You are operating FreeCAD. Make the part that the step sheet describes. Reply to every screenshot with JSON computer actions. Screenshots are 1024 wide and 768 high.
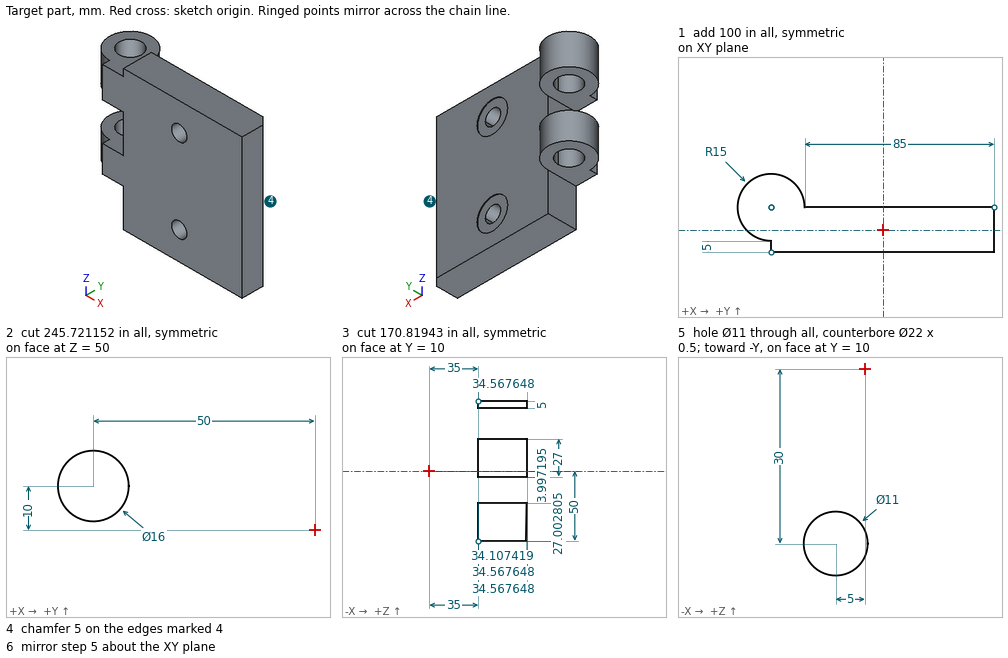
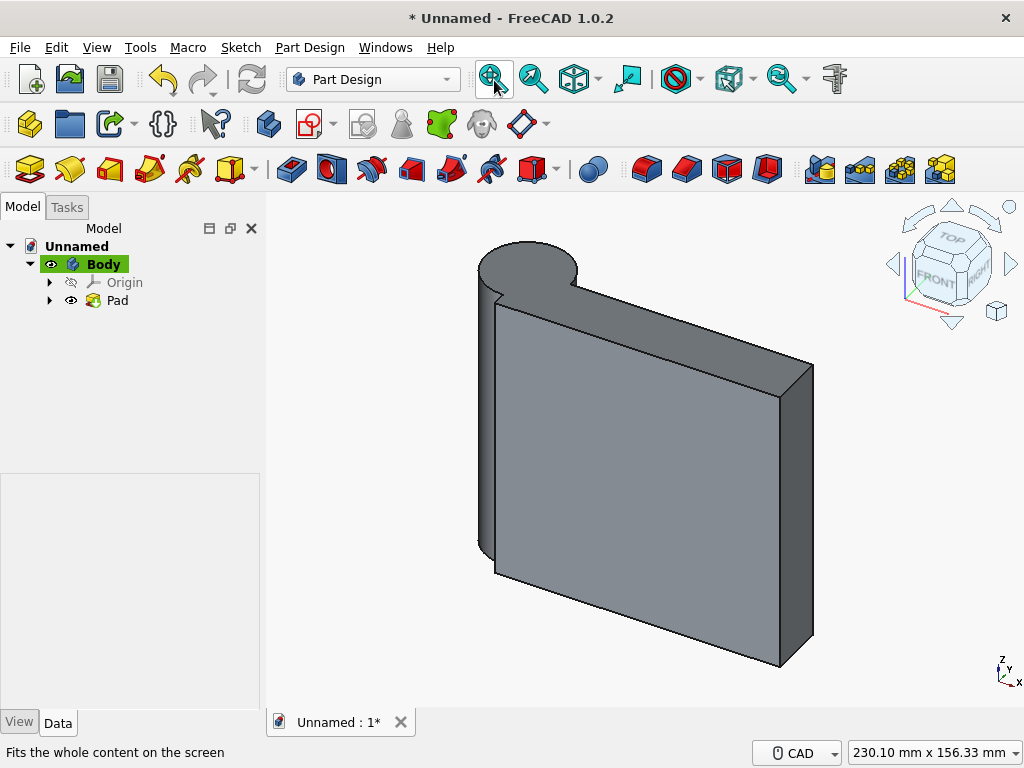
{"action": "left_click", "coordinate": [543, 291]}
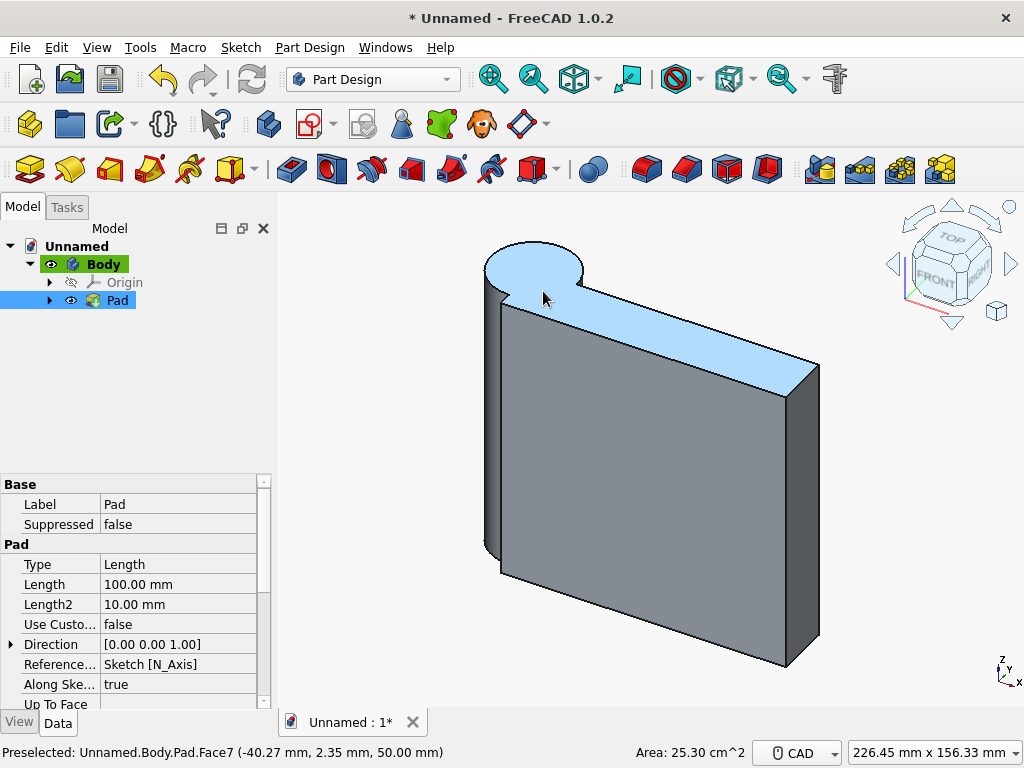
{"action": "left_click", "coordinate": [310, 124]}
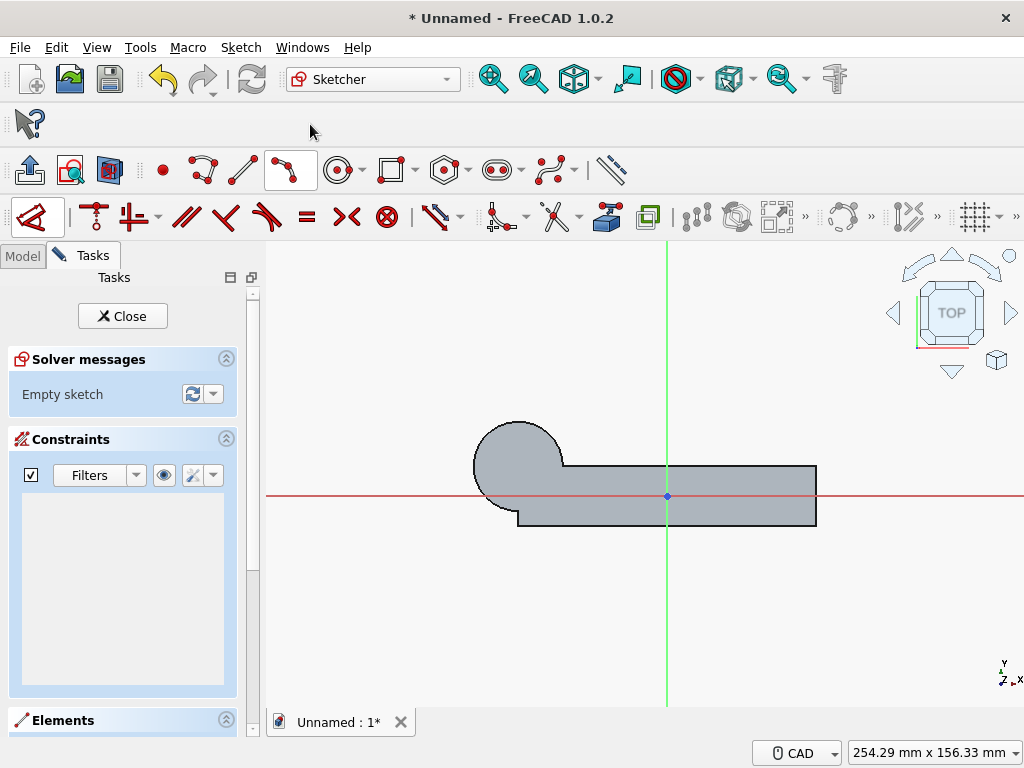
{"action": "scroll", "coordinate": [507, 465], "scroll_direction": "up", "scroll_amount": 9}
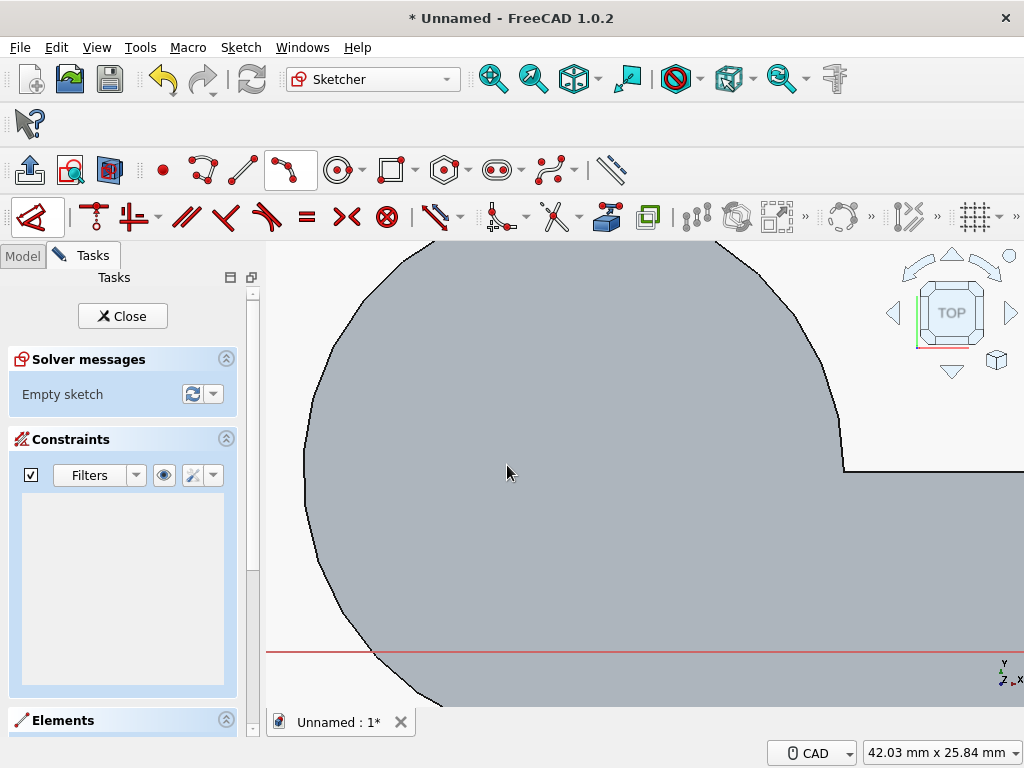
{"action": "left_click", "coordinate": [338, 170]}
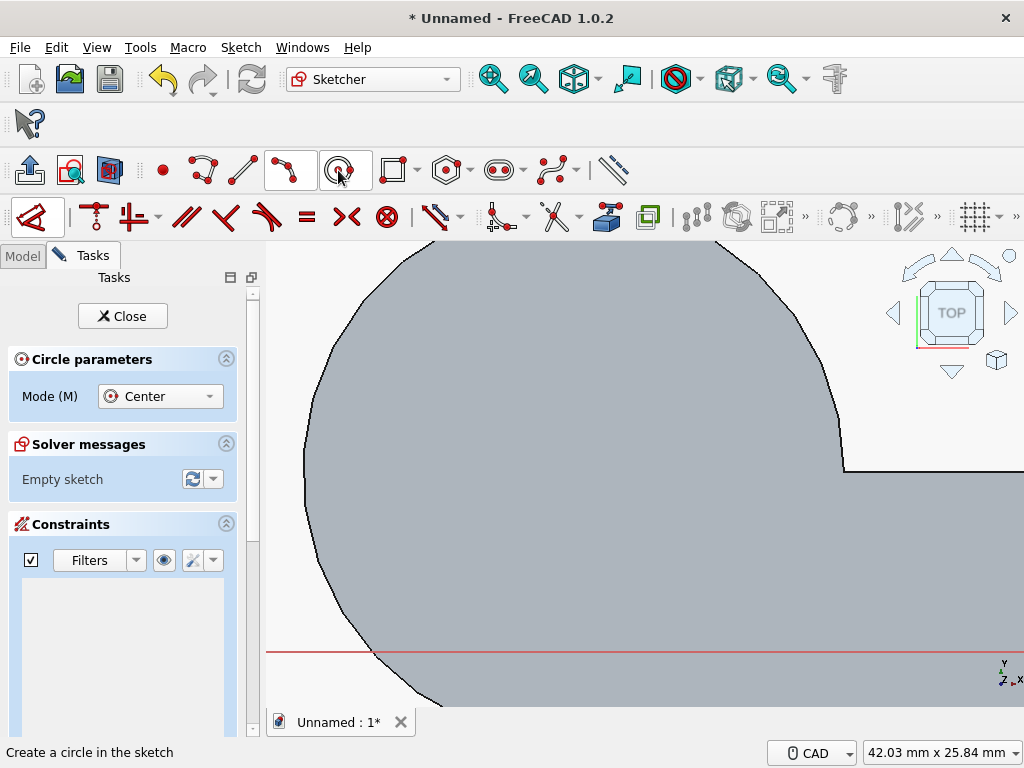
{"action": "left_click", "coordinate": [574, 472]}
{"action": "mouse_move", "coordinate": [676, 370]}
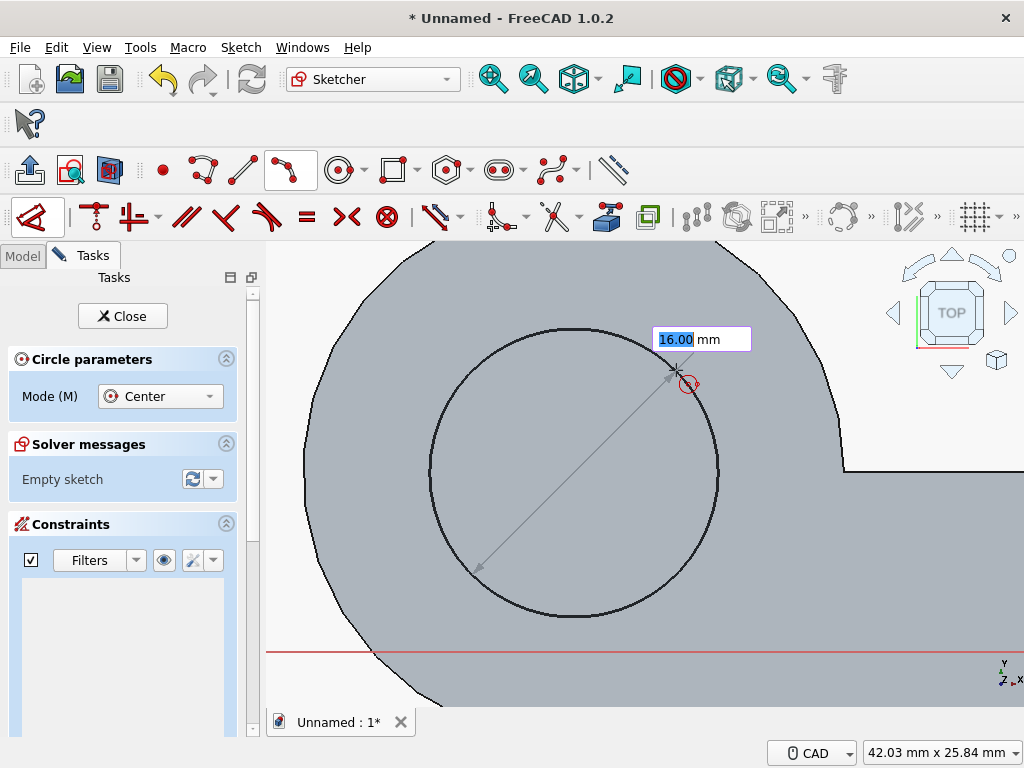
{"action": "type", "text": "16"}
{"action": "key", "text": "Return"}
{"action": "key", "text": "Escape"}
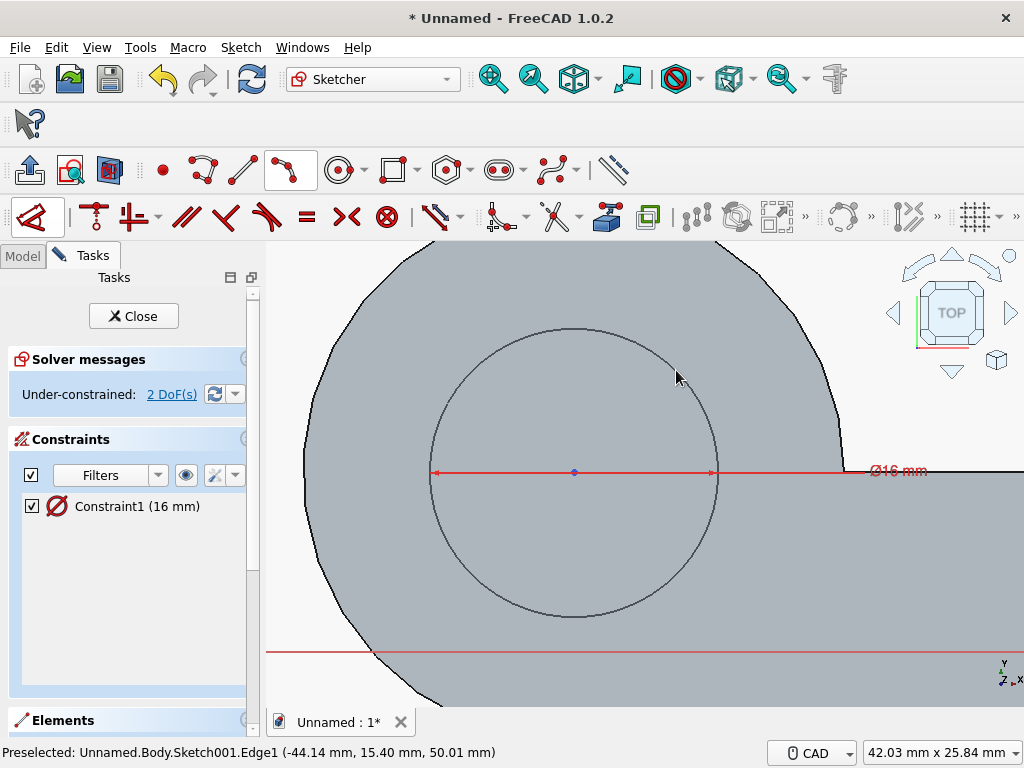
{"action": "left_click", "coordinate": [574, 473]}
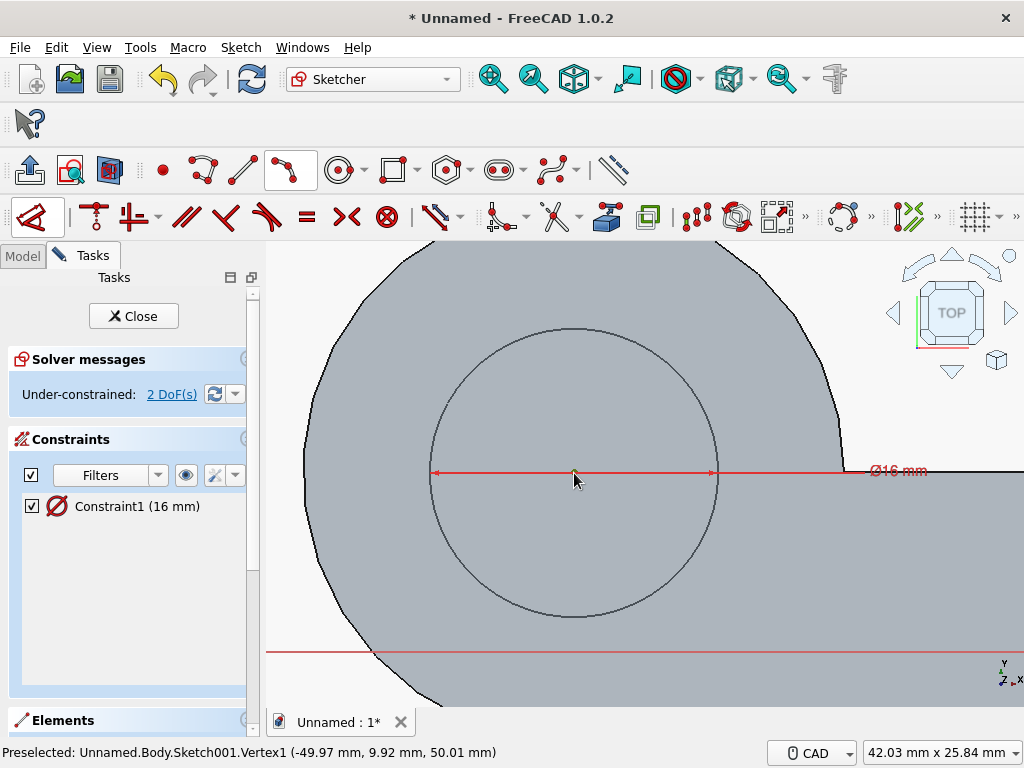
{"action": "key", "text": "l"}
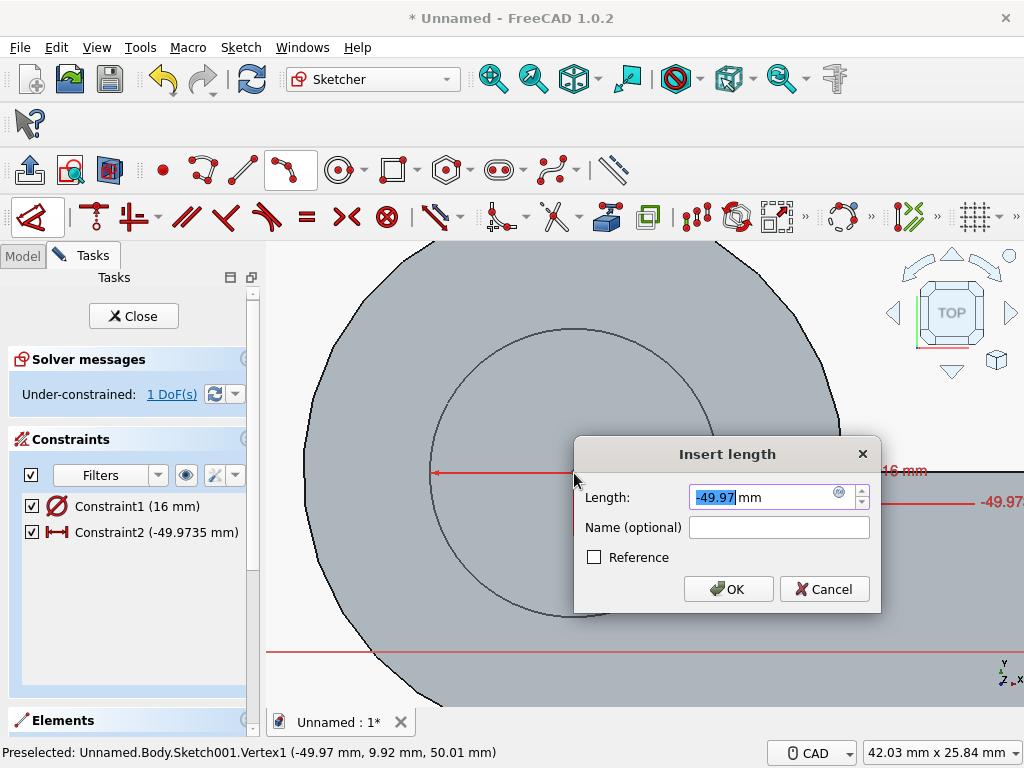
{"action": "type", "text": "-50"}
{"action": "key", "text": "Return"}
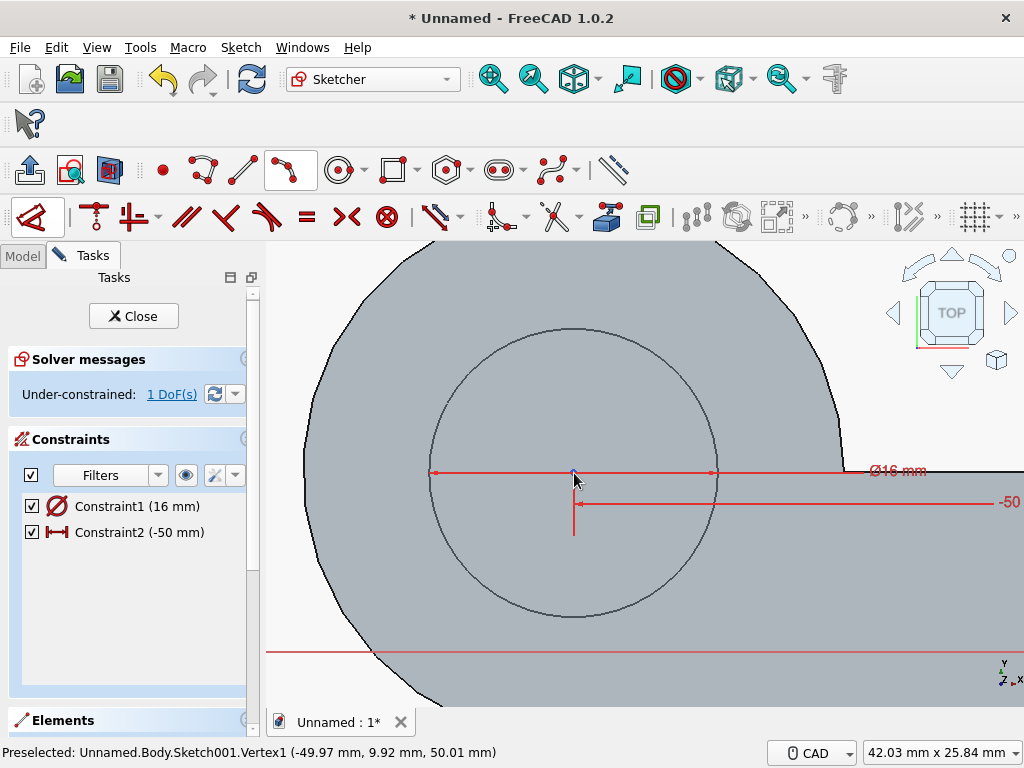
{"action": "left_click", "coordinate": [574, 473]}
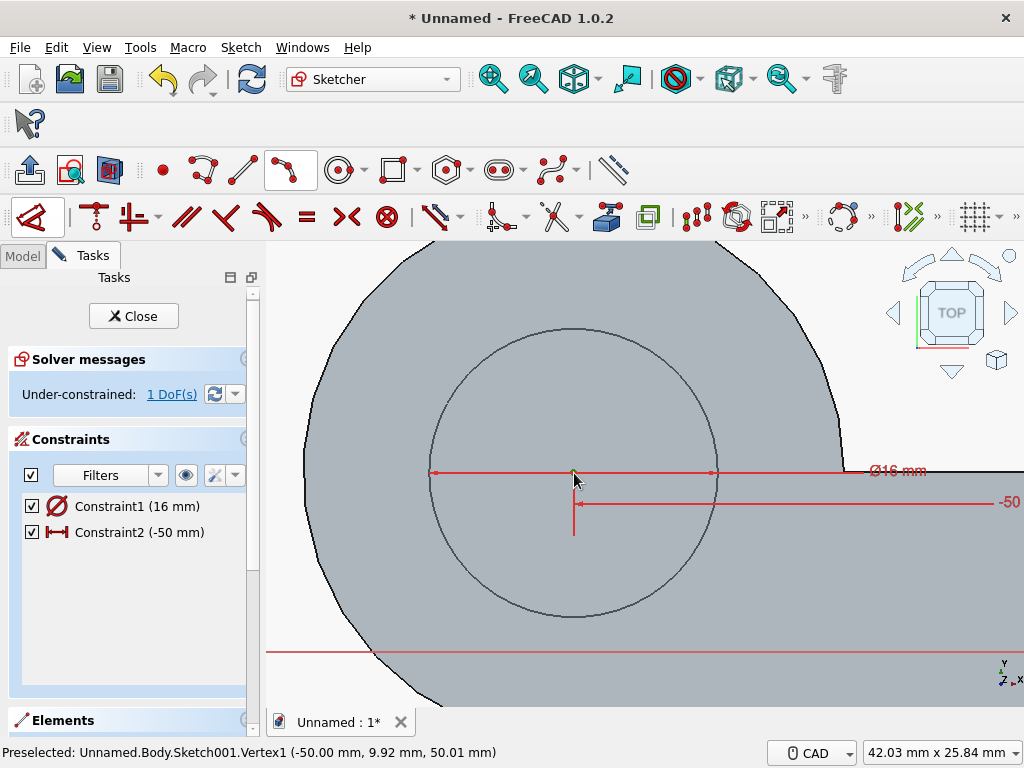
{"action": "key", "text": "i"}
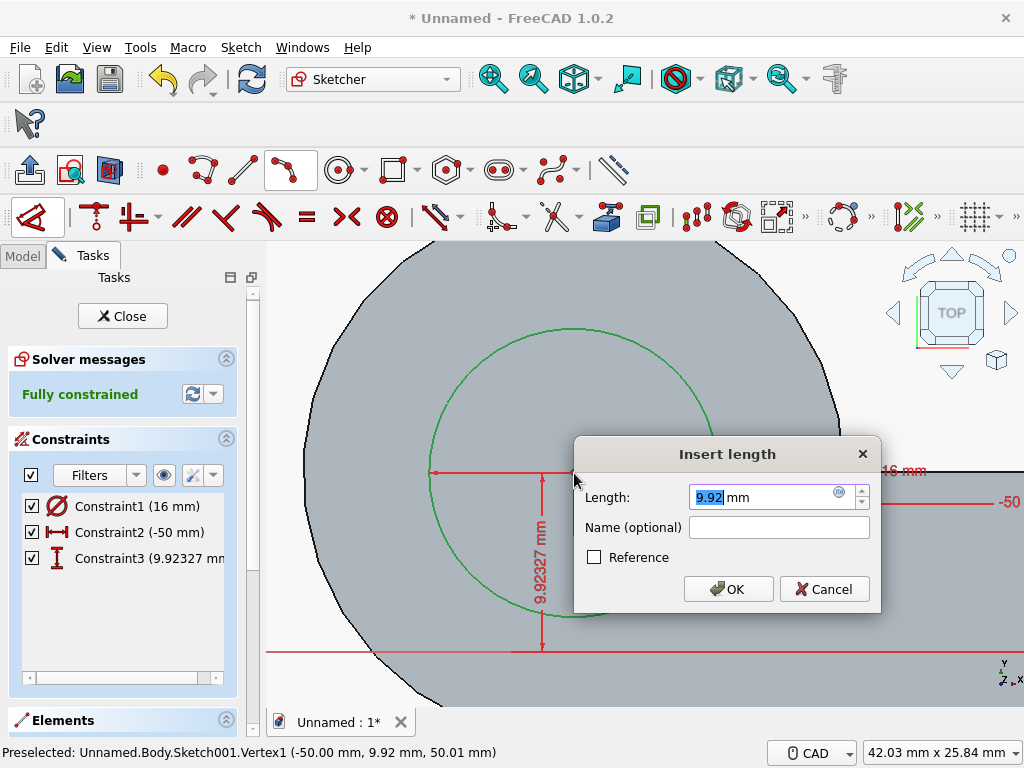
{"action": "type", "text": "10"}
{"action": "key", "text": "Return"}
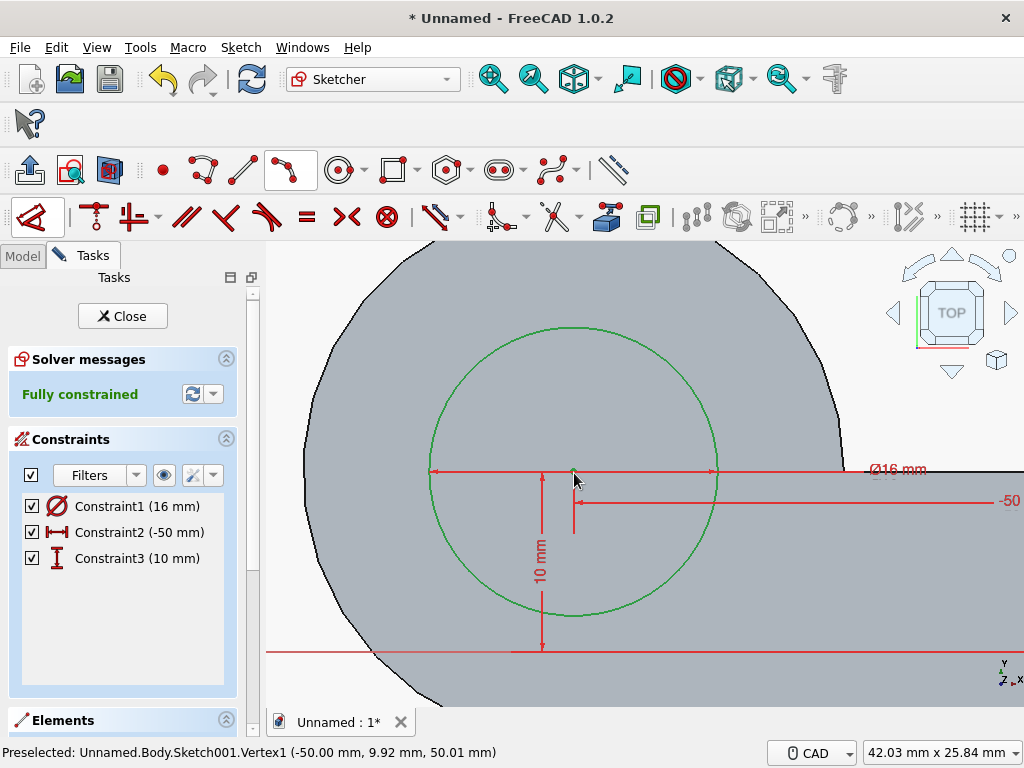
{"action": "left_click", "coordinate": [123, 316]}